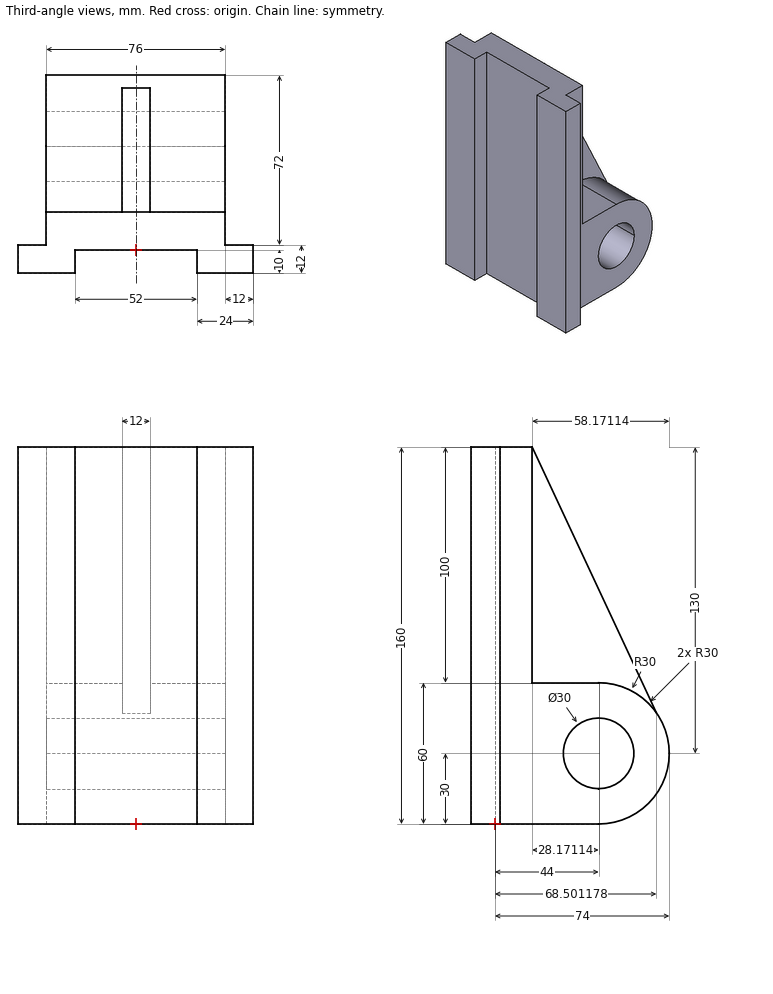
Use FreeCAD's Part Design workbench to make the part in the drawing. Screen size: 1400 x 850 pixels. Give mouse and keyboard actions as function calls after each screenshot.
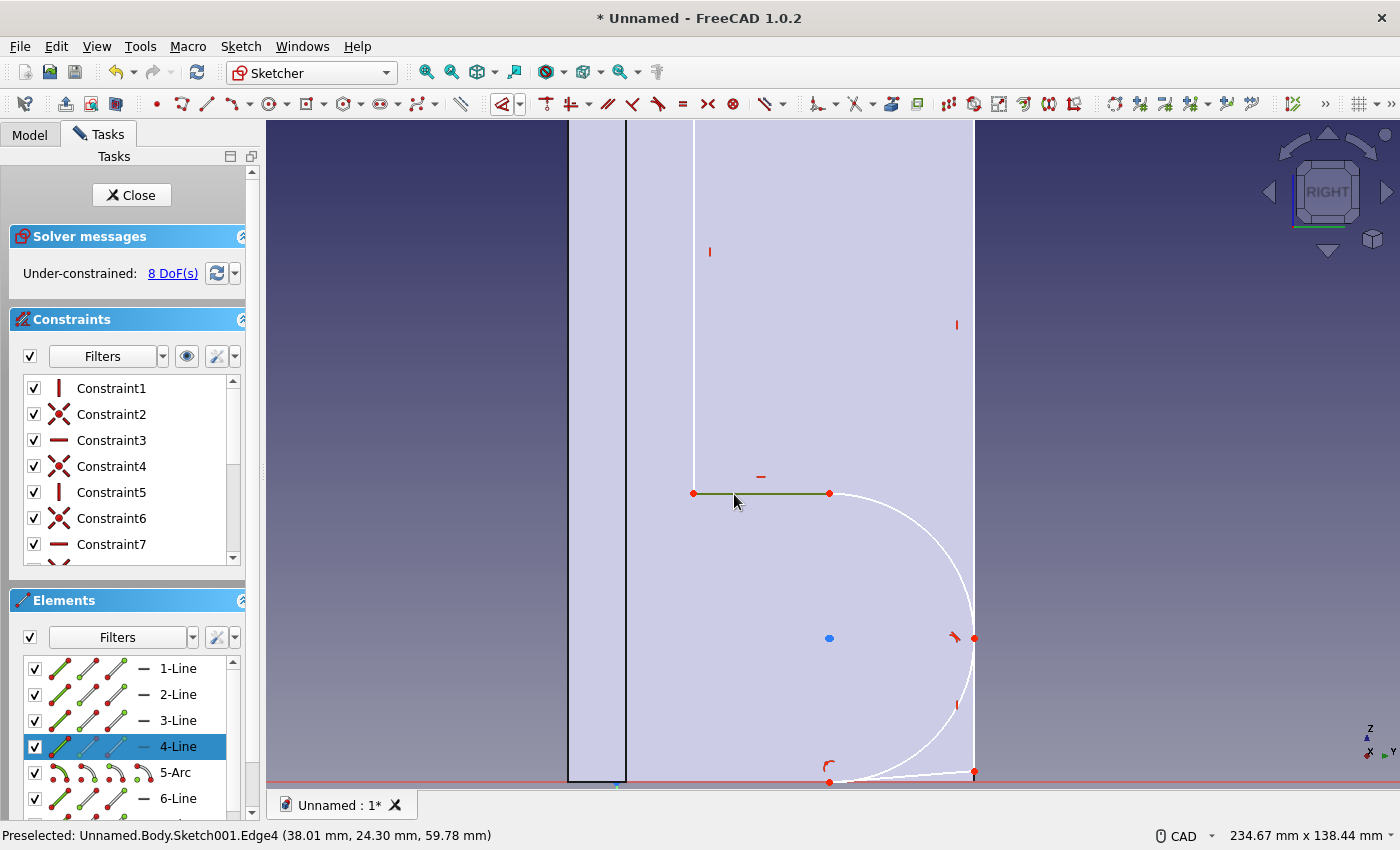
click(958, 573)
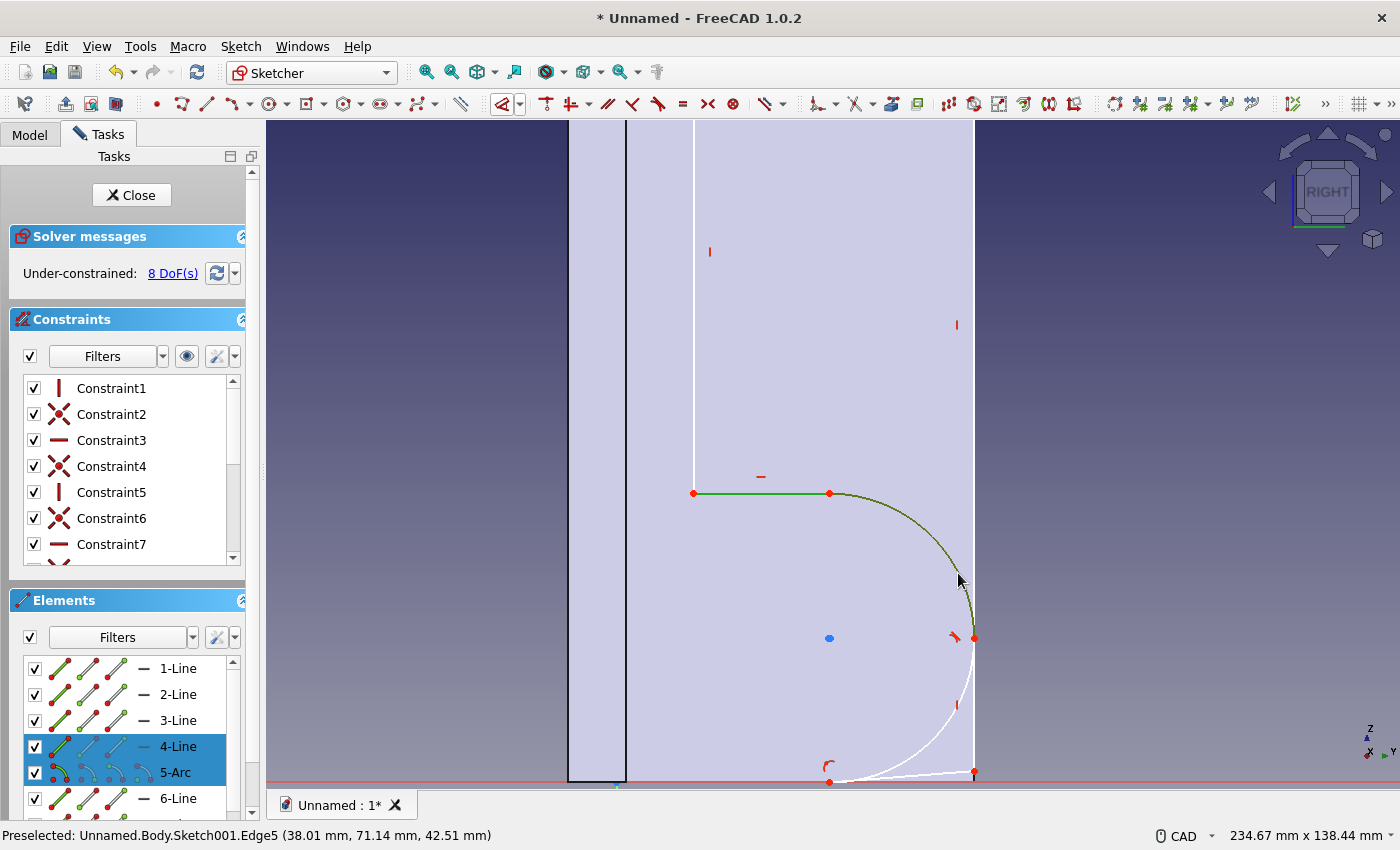
key(t)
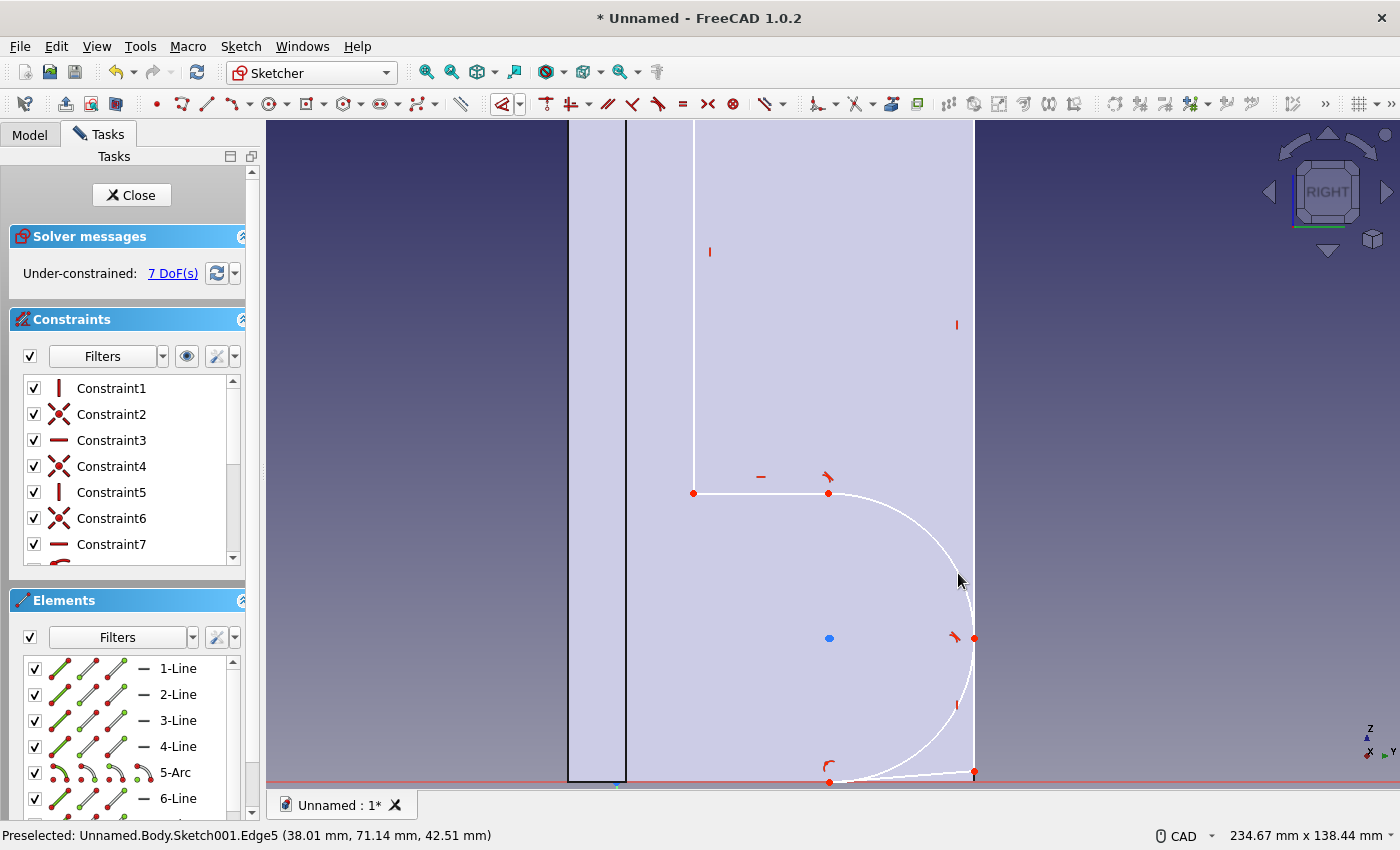
scroll(727, 526, down, 3)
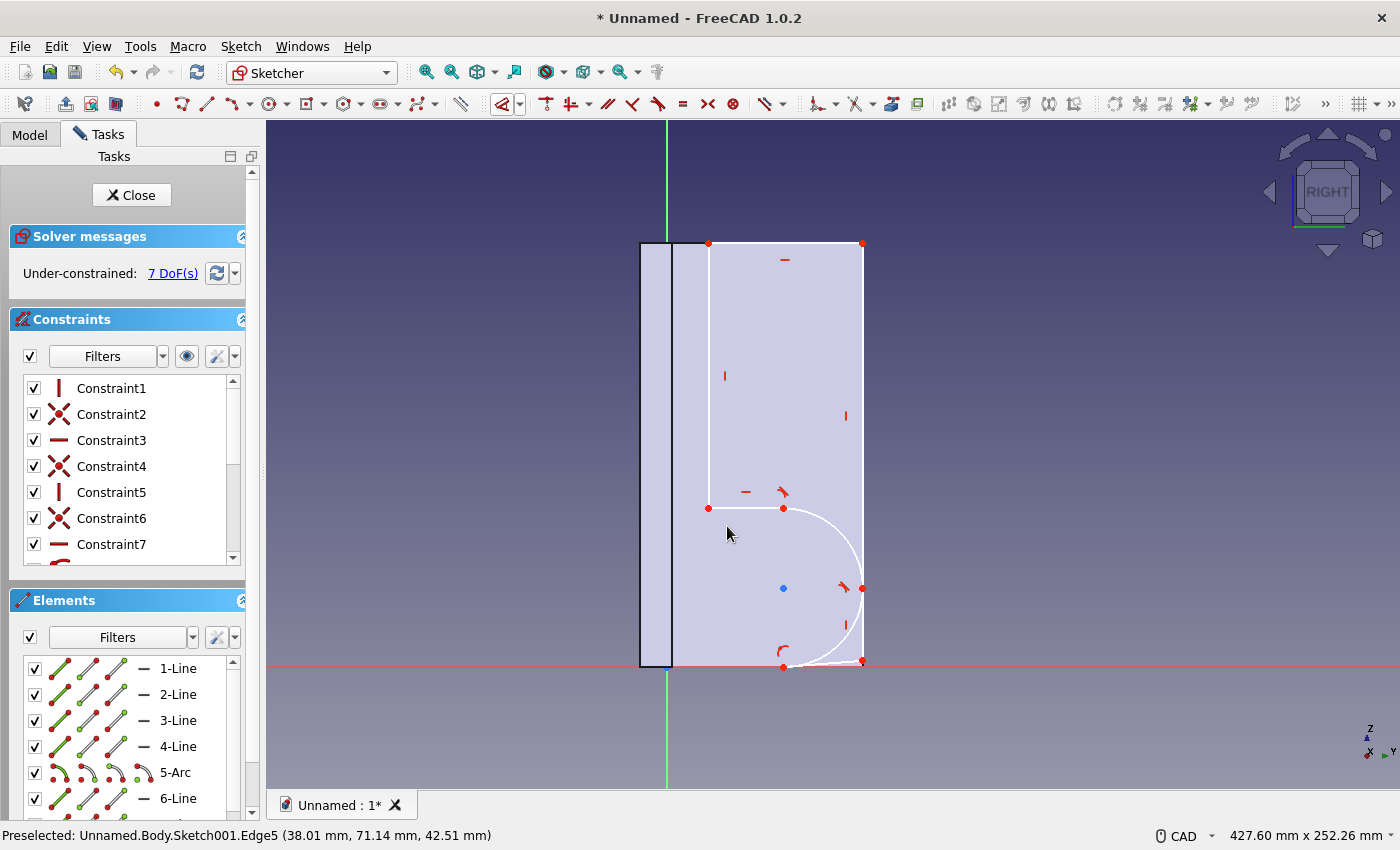
scroll(847, 662, up, 6)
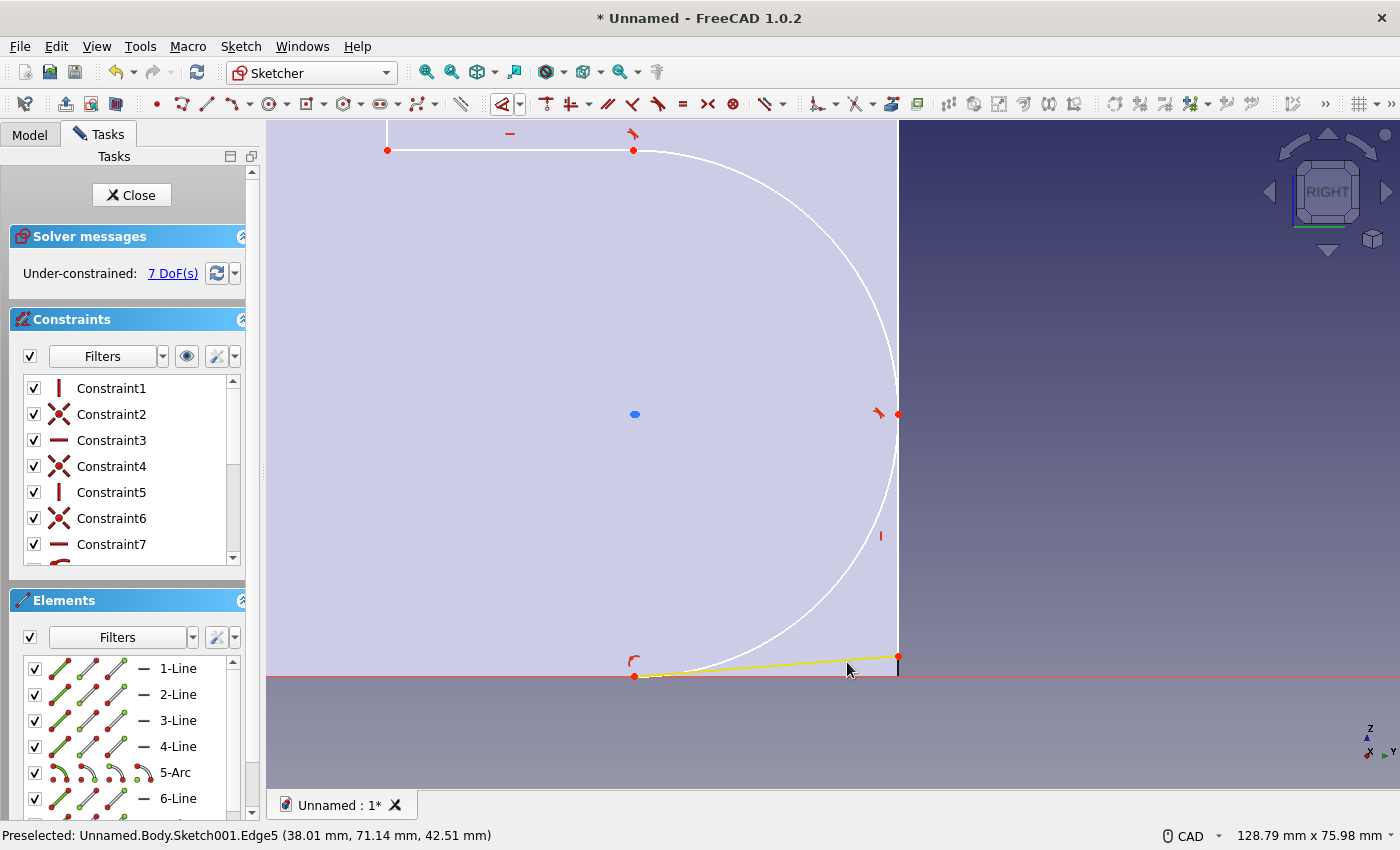
click(846, 660)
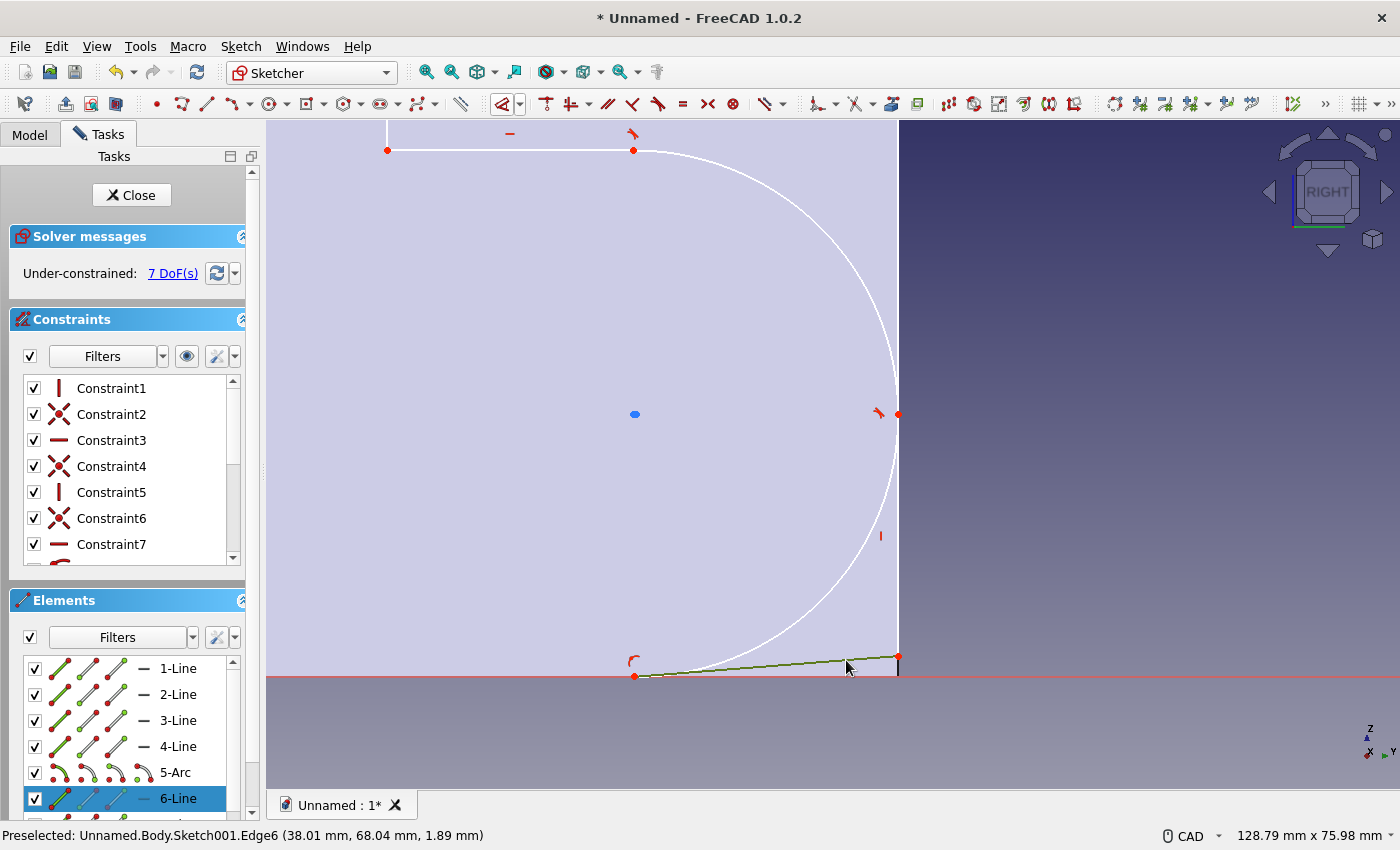
click(754, 649)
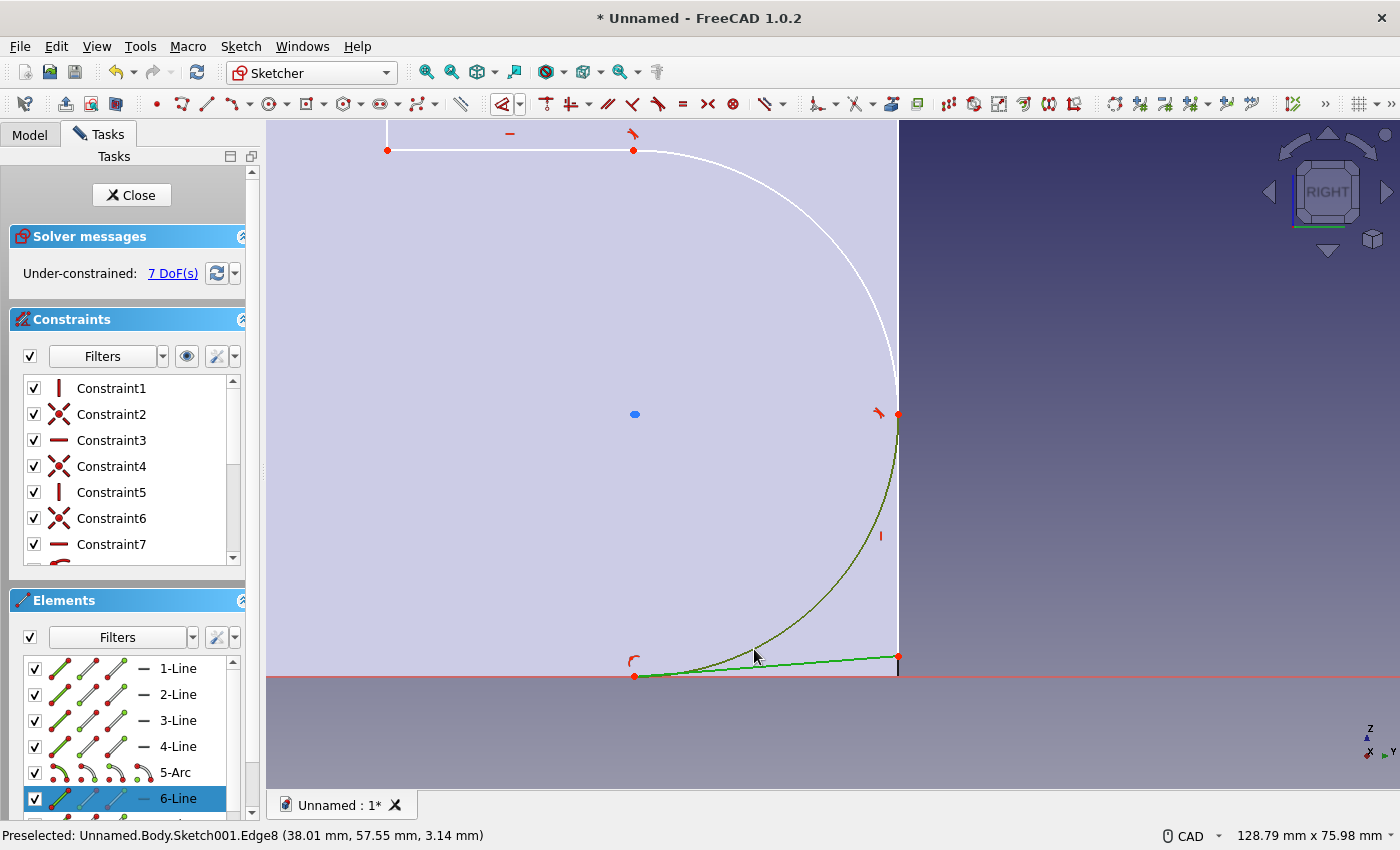
click(658, 104)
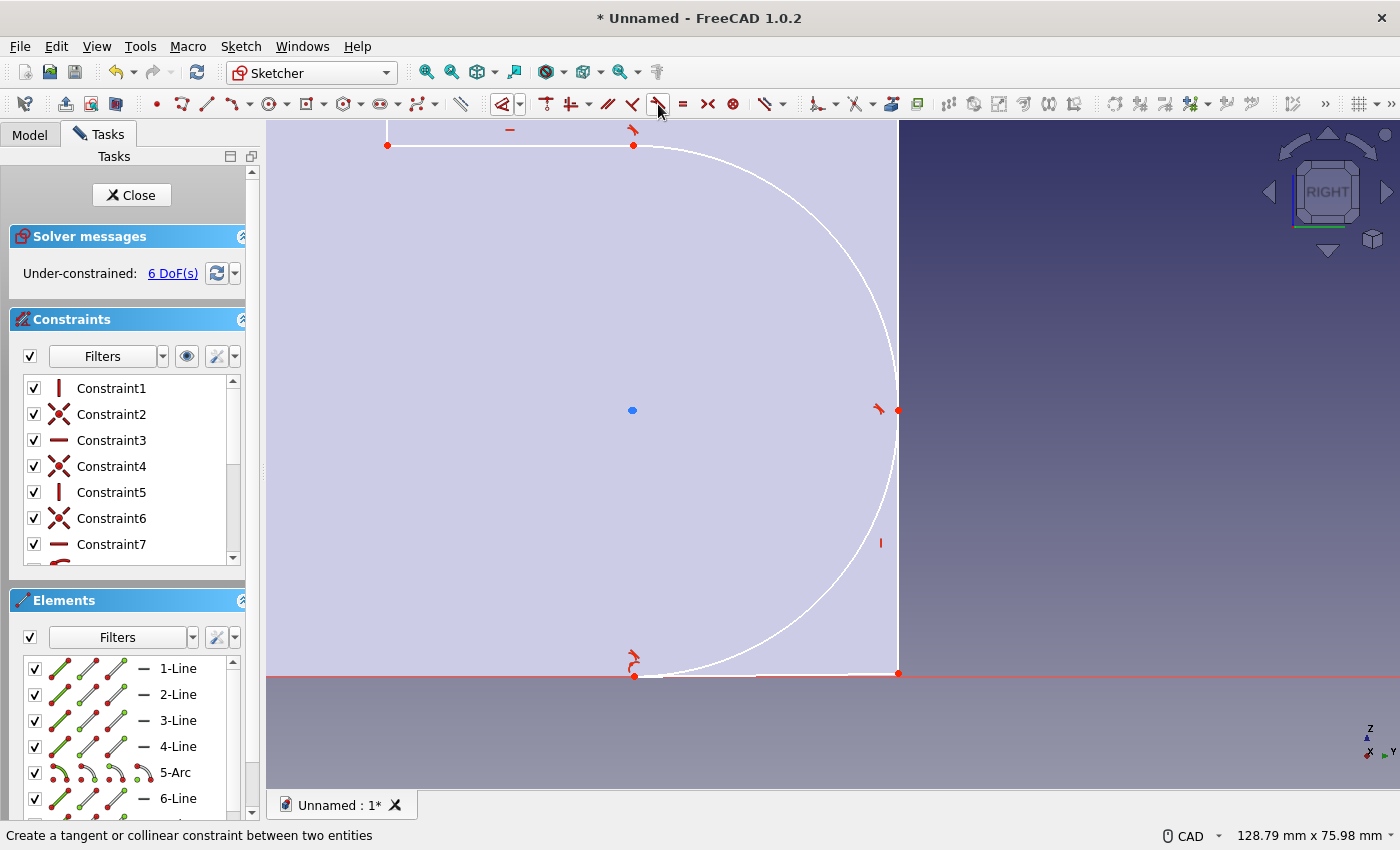
click(714, 676)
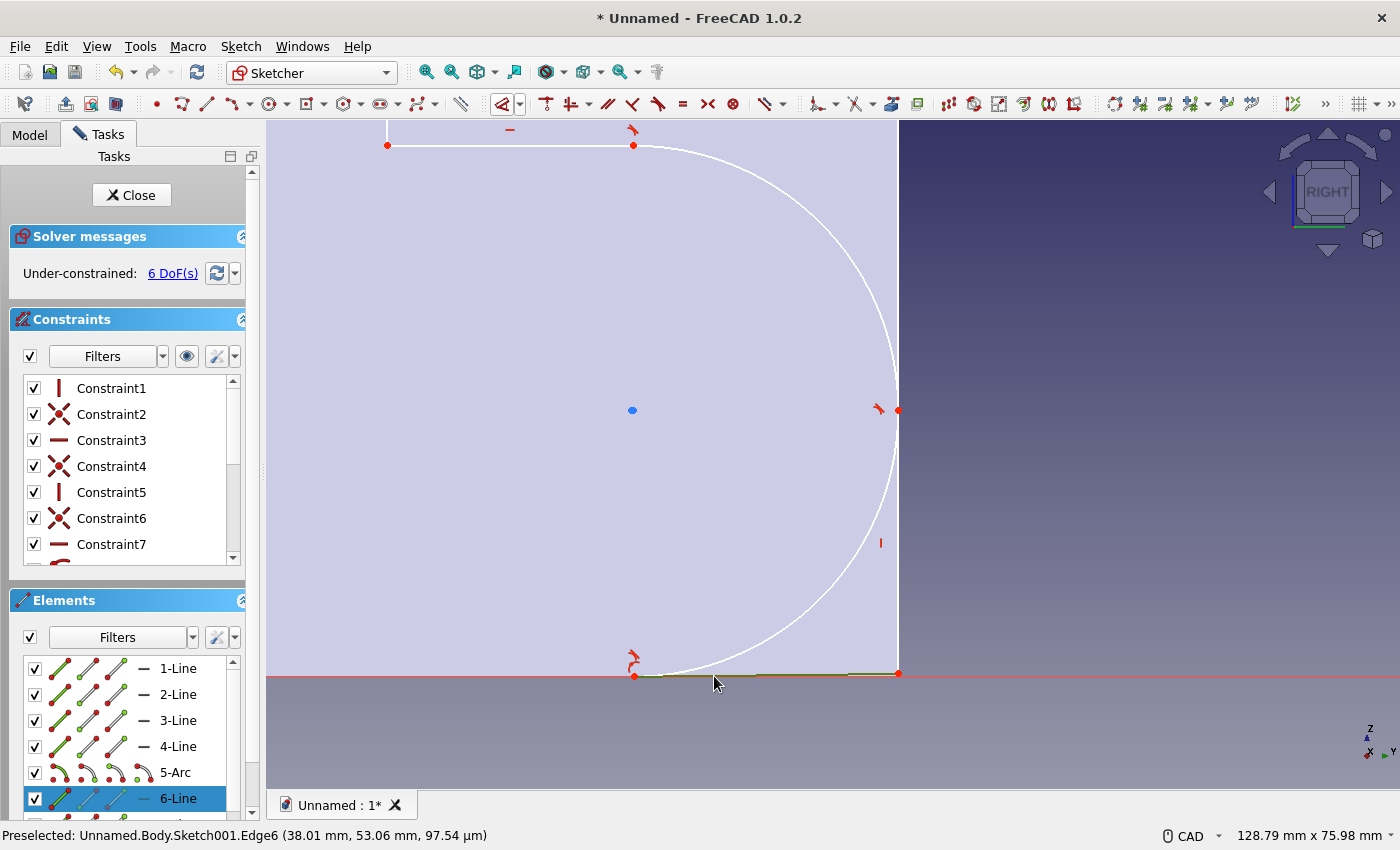
click(588, 104)